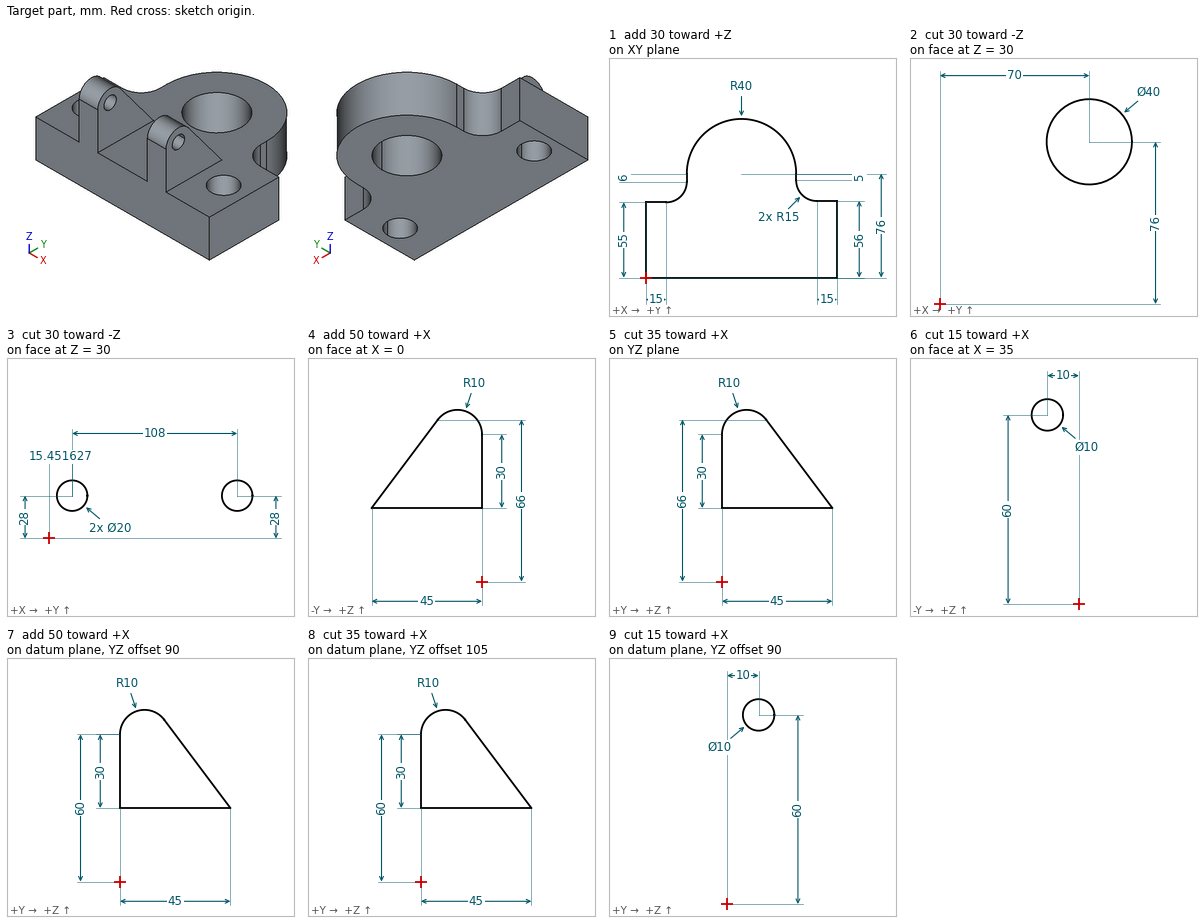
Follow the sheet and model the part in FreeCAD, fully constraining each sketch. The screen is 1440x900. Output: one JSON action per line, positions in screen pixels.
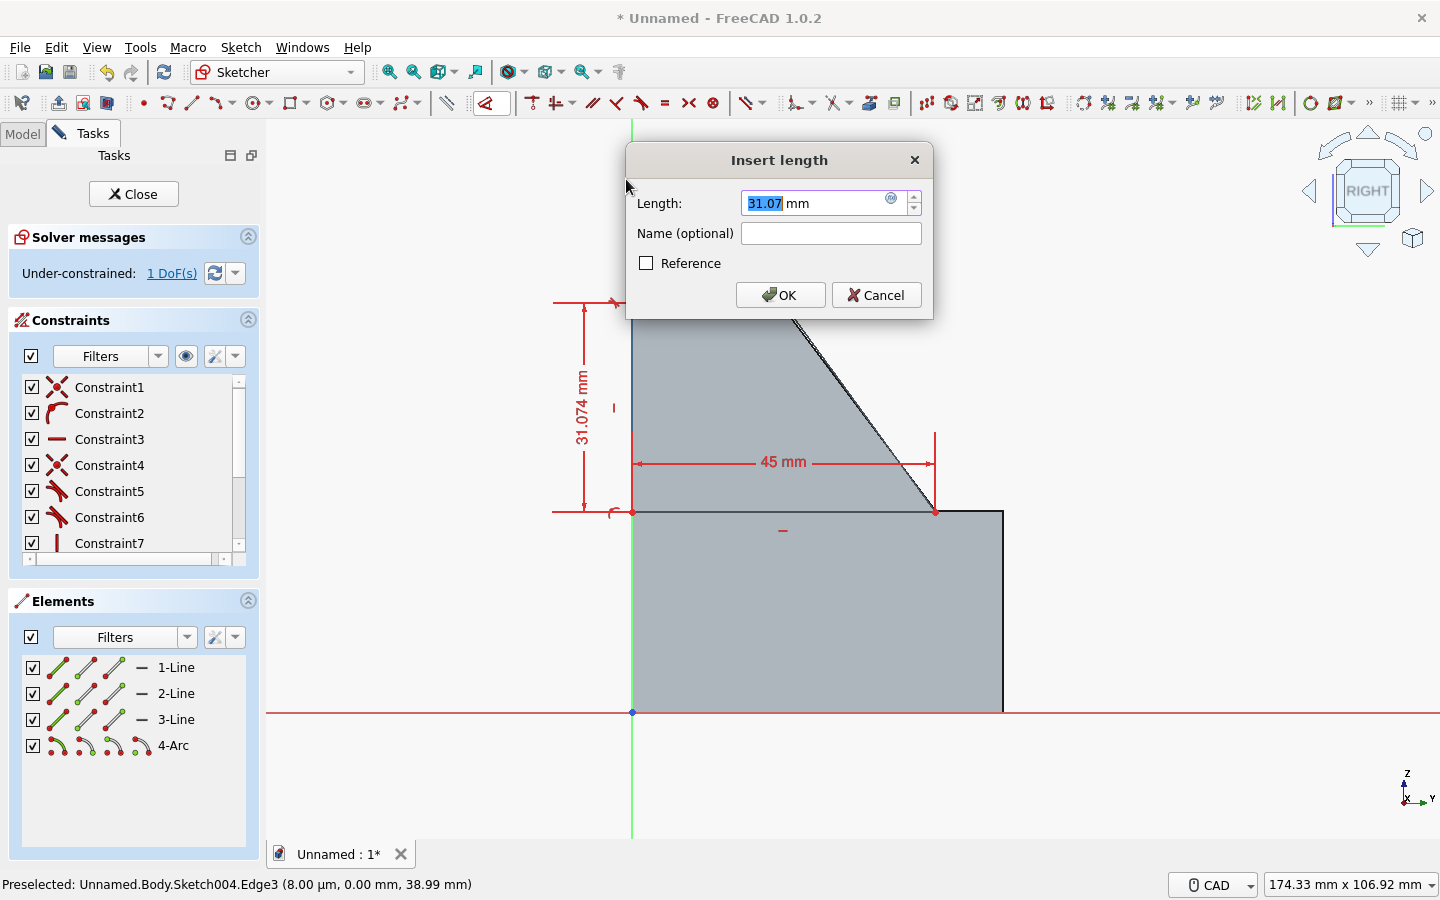
{"action": "type", "text": "30"}
{"action": "key", "text": "Return"}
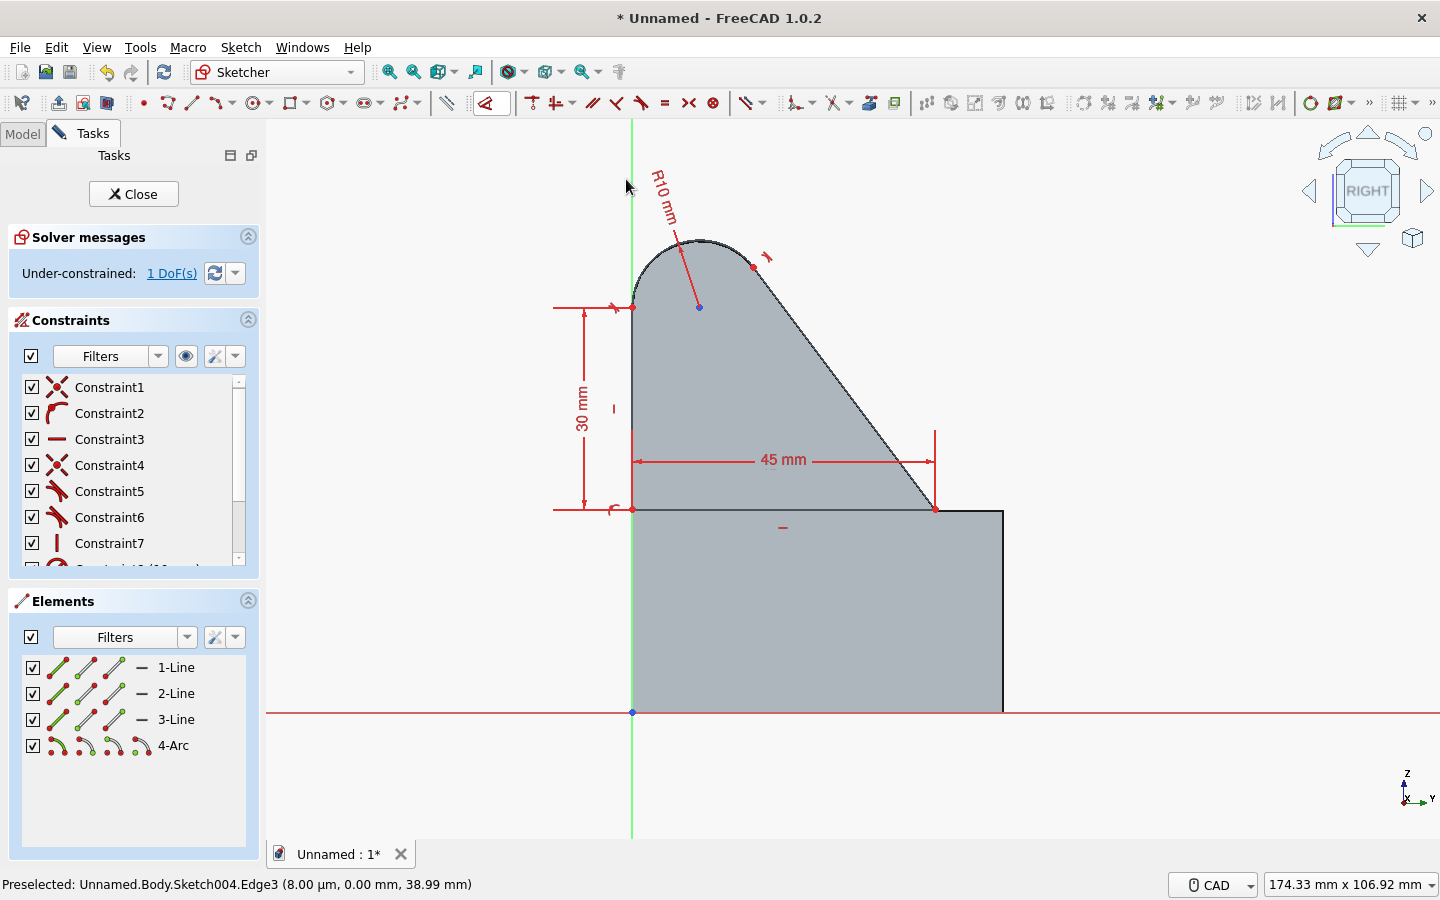
{"action": "left_click", "coordinate": [754, 267]}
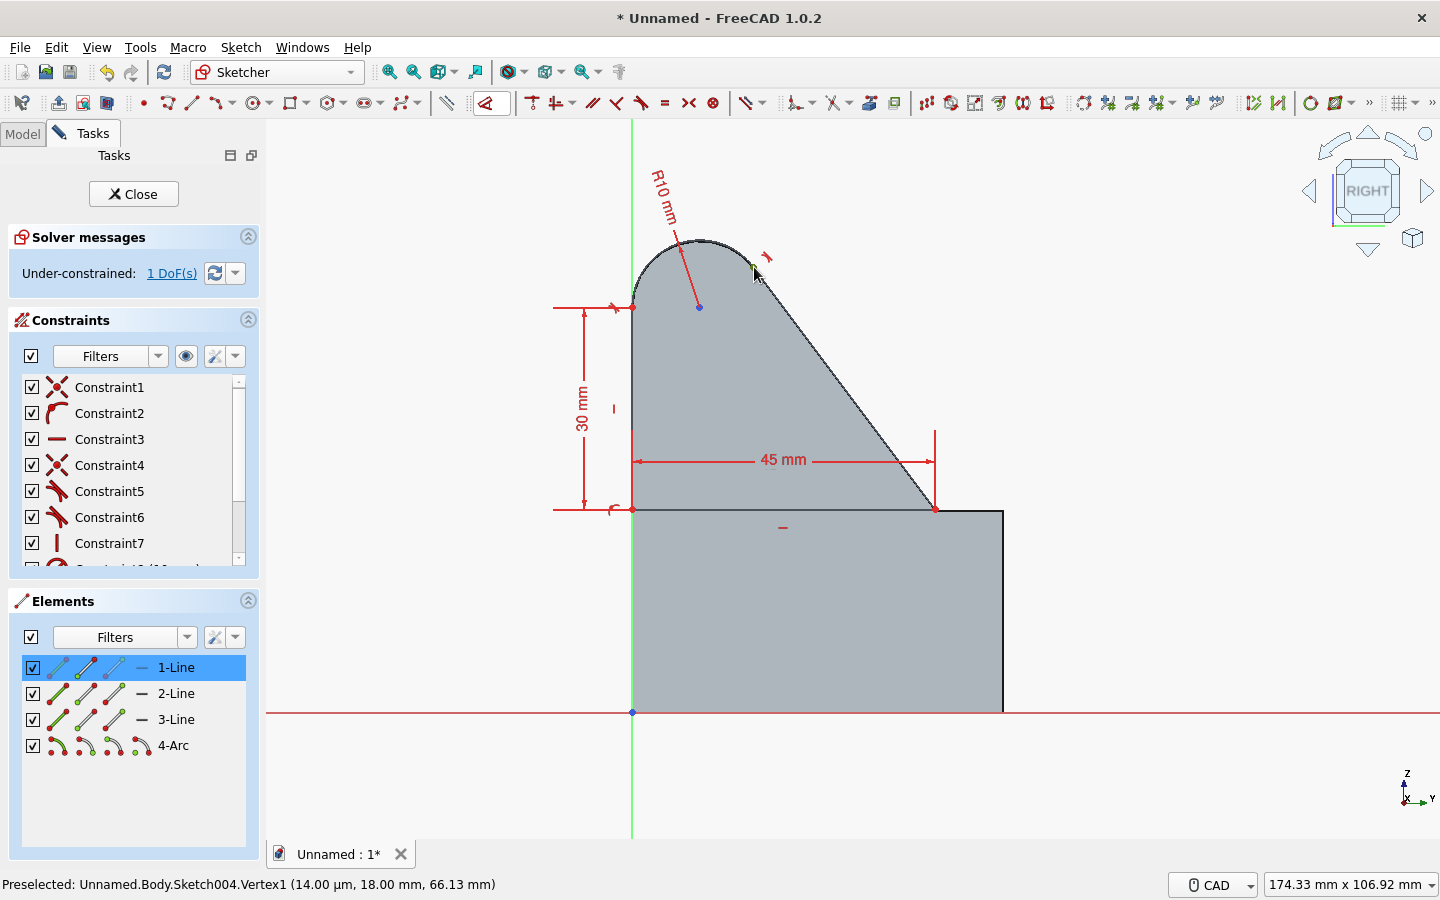
{"action": "left_click", "coordinate": [504, 104]}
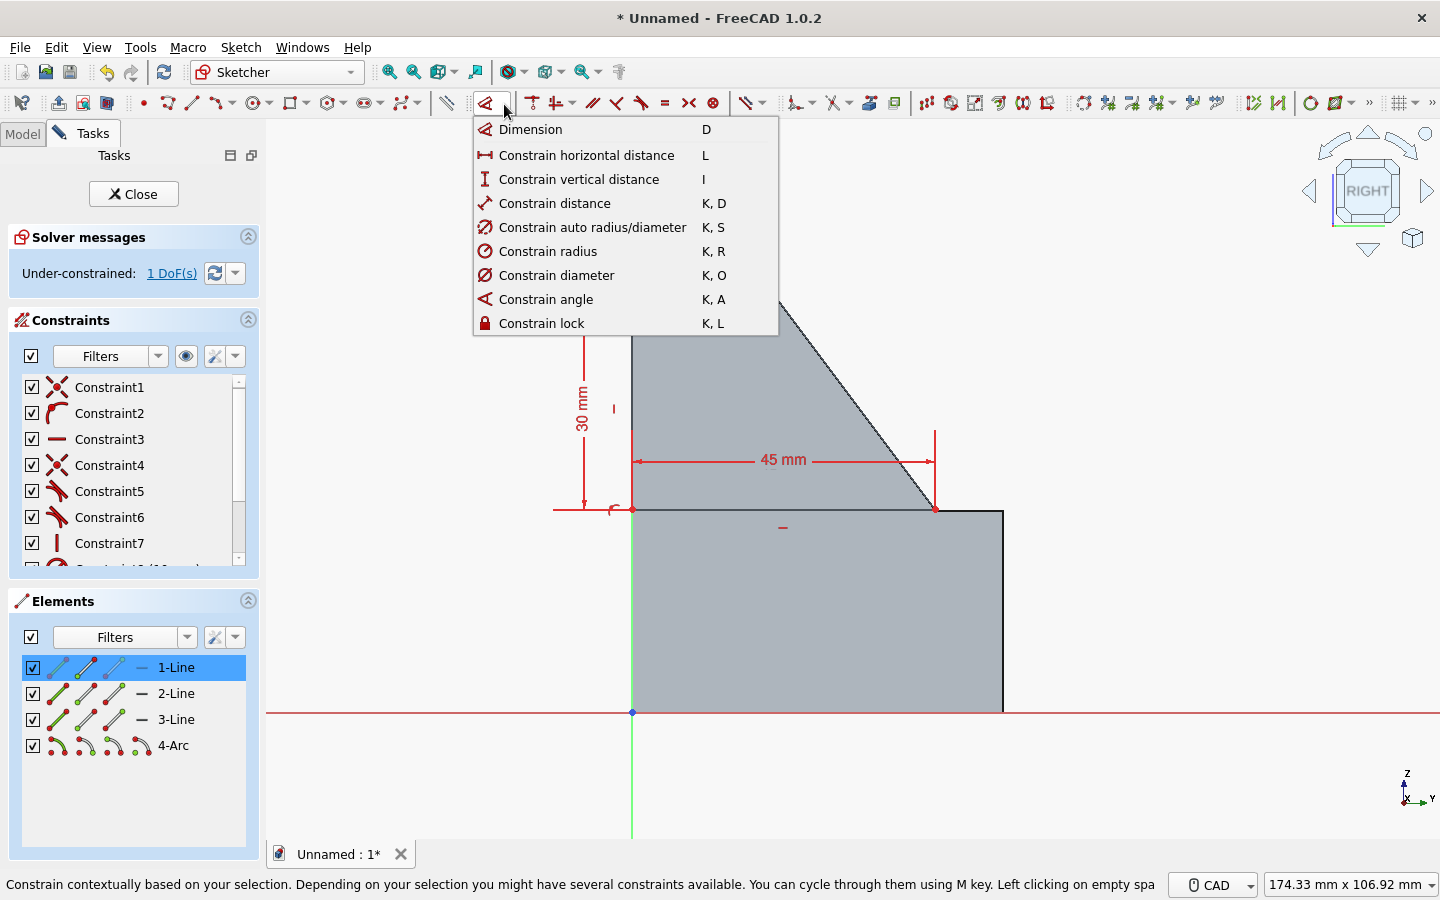
{"action": "left_click", "coordinate": [626, 179]}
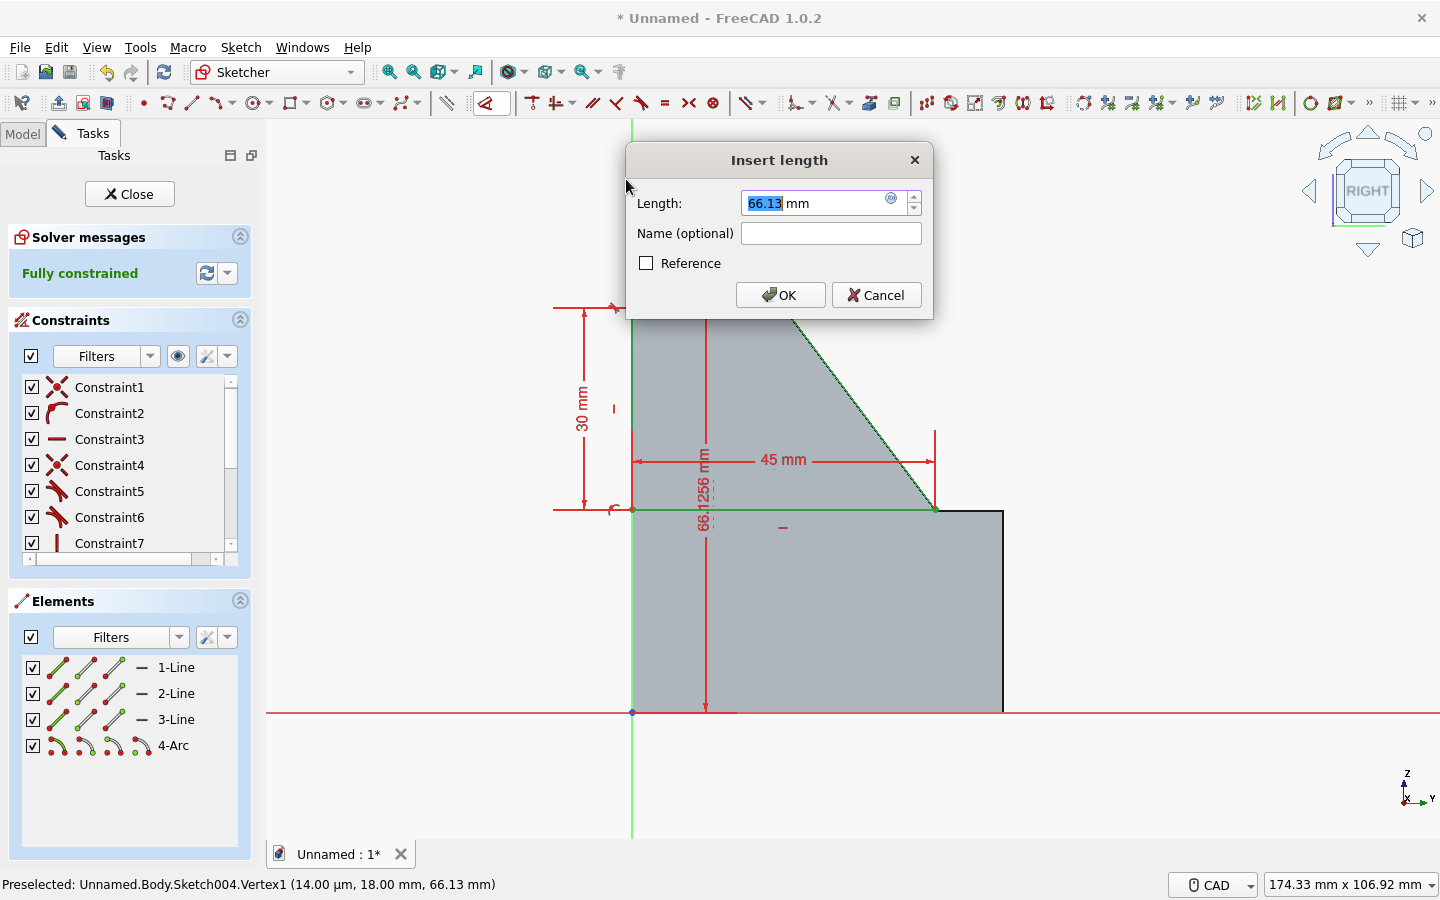
{"action": "type", "text": "66"}
{"action": "key", "text": "Return"}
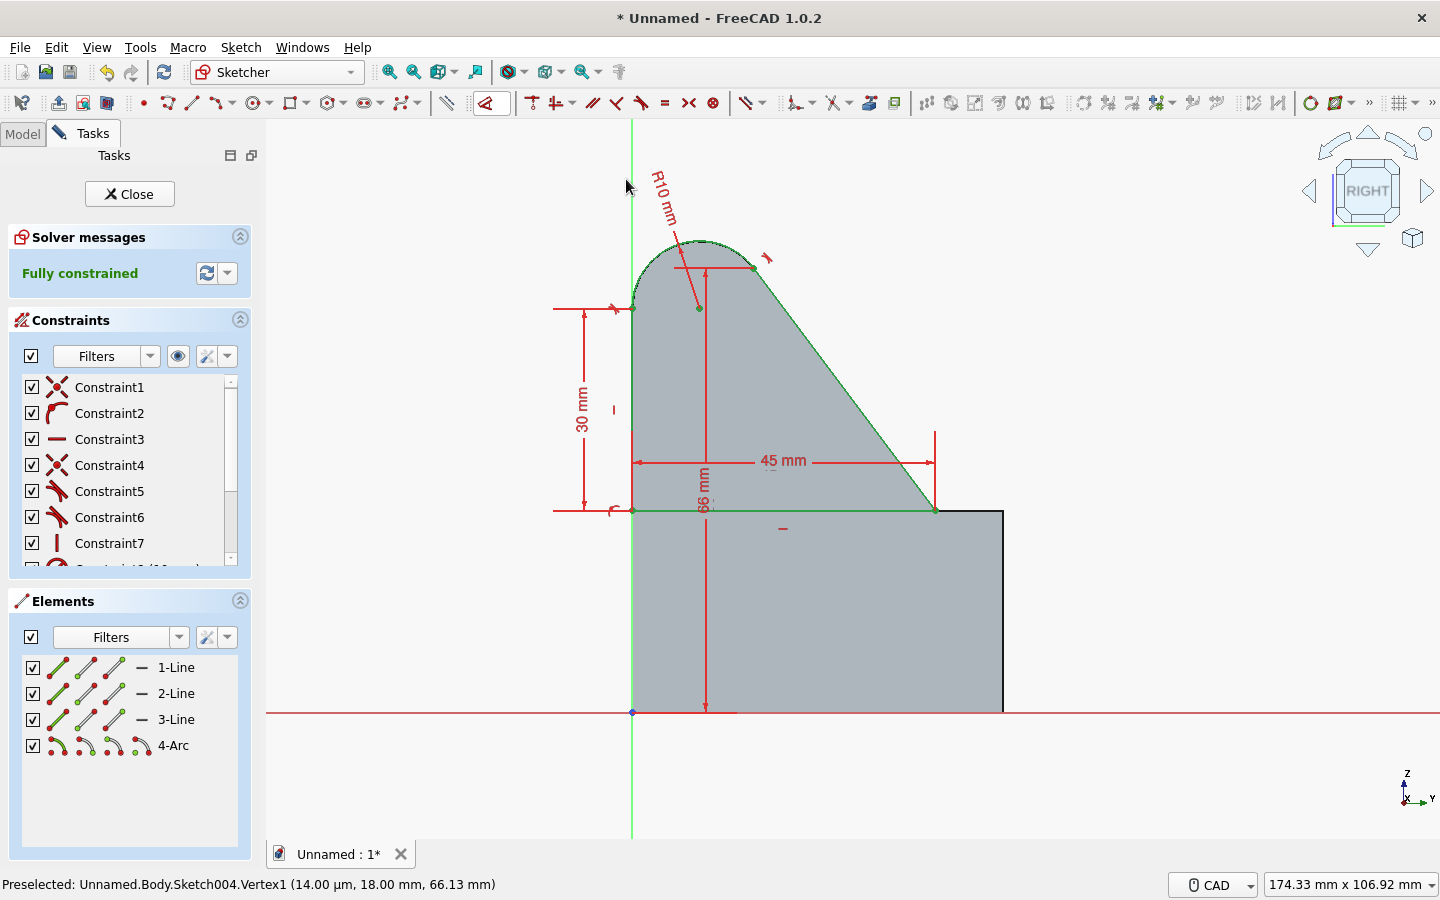
{"action": "left_click", "coordinate": [130, 194]}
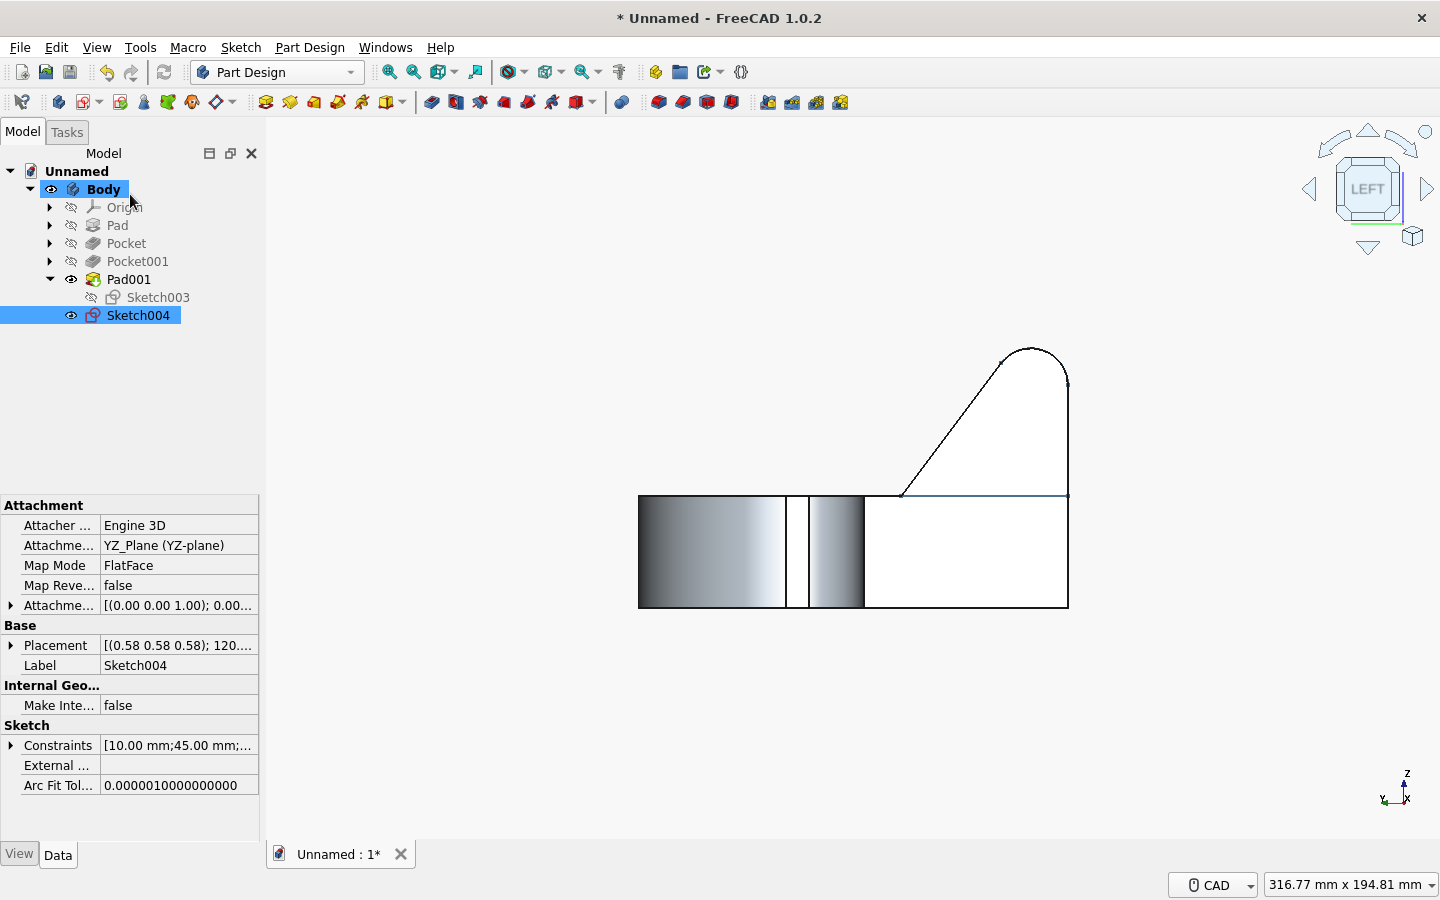
{"action": "left_click", "coordinate": [432, 102]}